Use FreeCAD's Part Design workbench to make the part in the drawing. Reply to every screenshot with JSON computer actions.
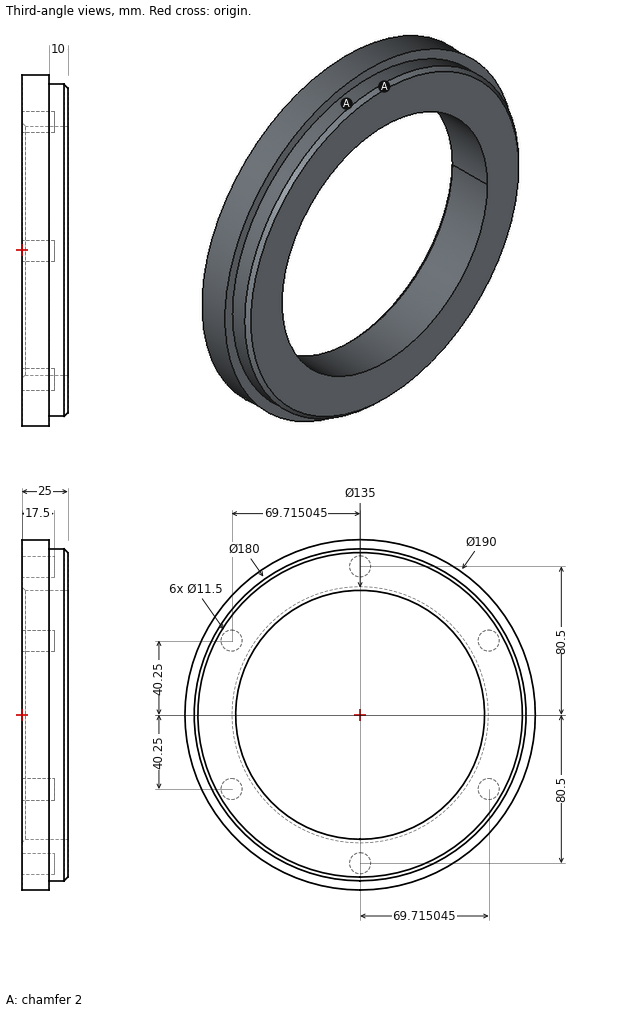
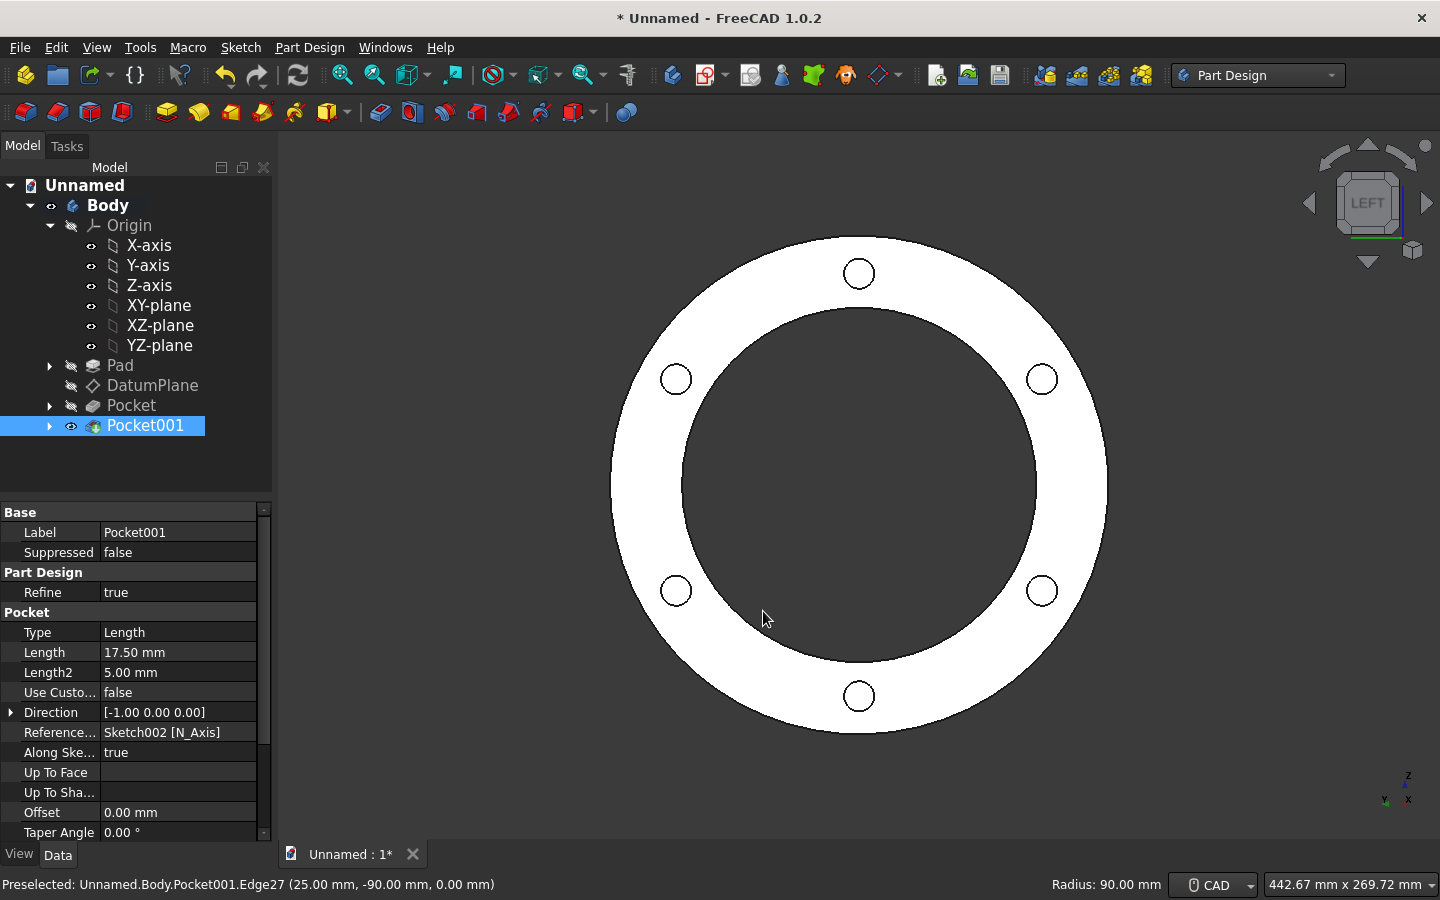
{"action": "left_click", "coordinate": [1036, 484], "text": "ctrl"}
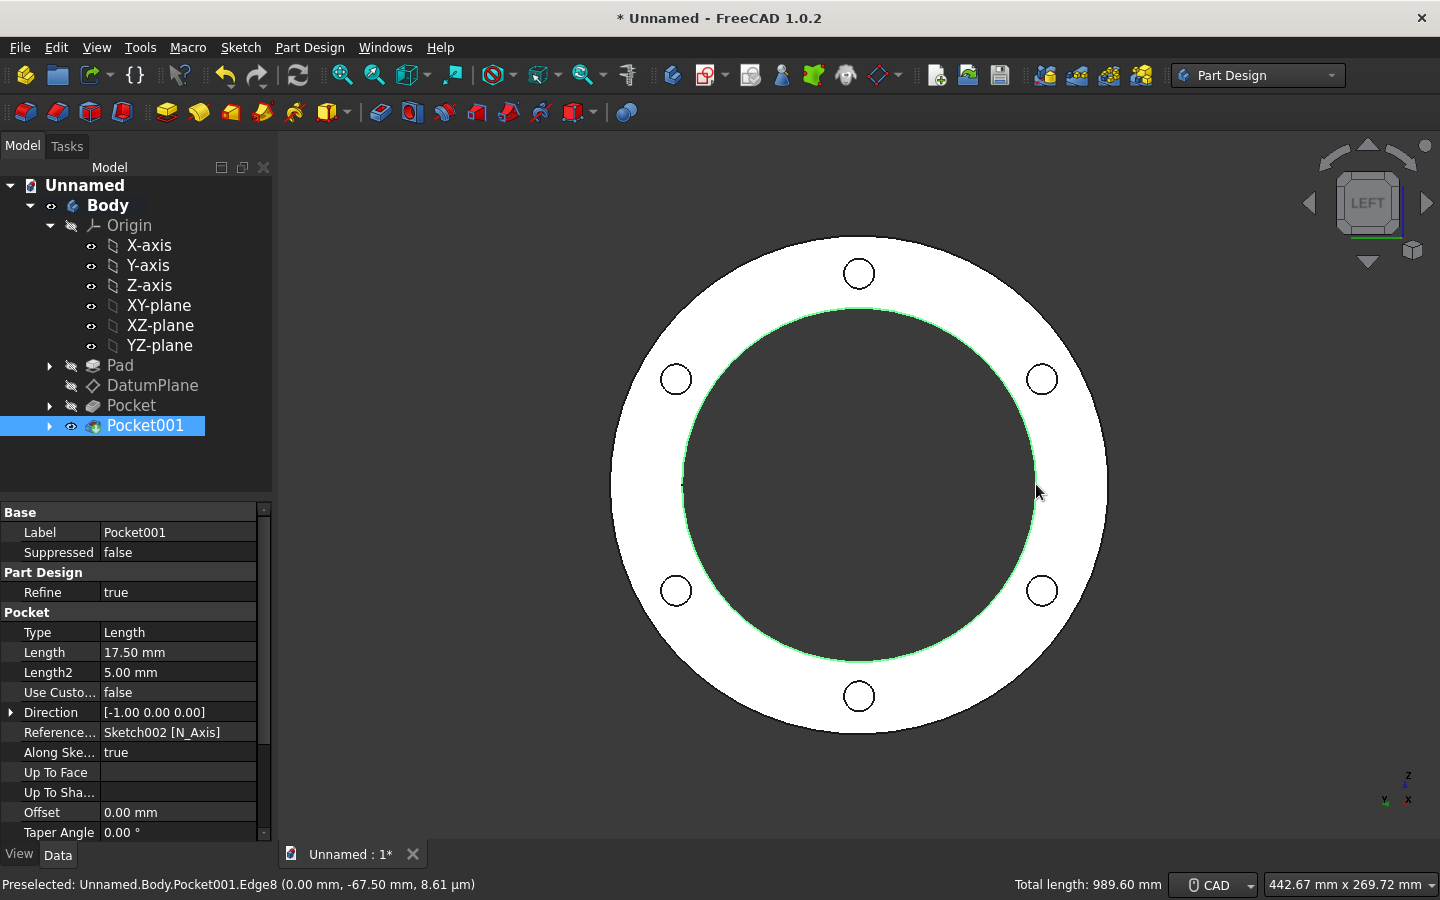
{"action": "left_click", "coordinate": [58, 112]}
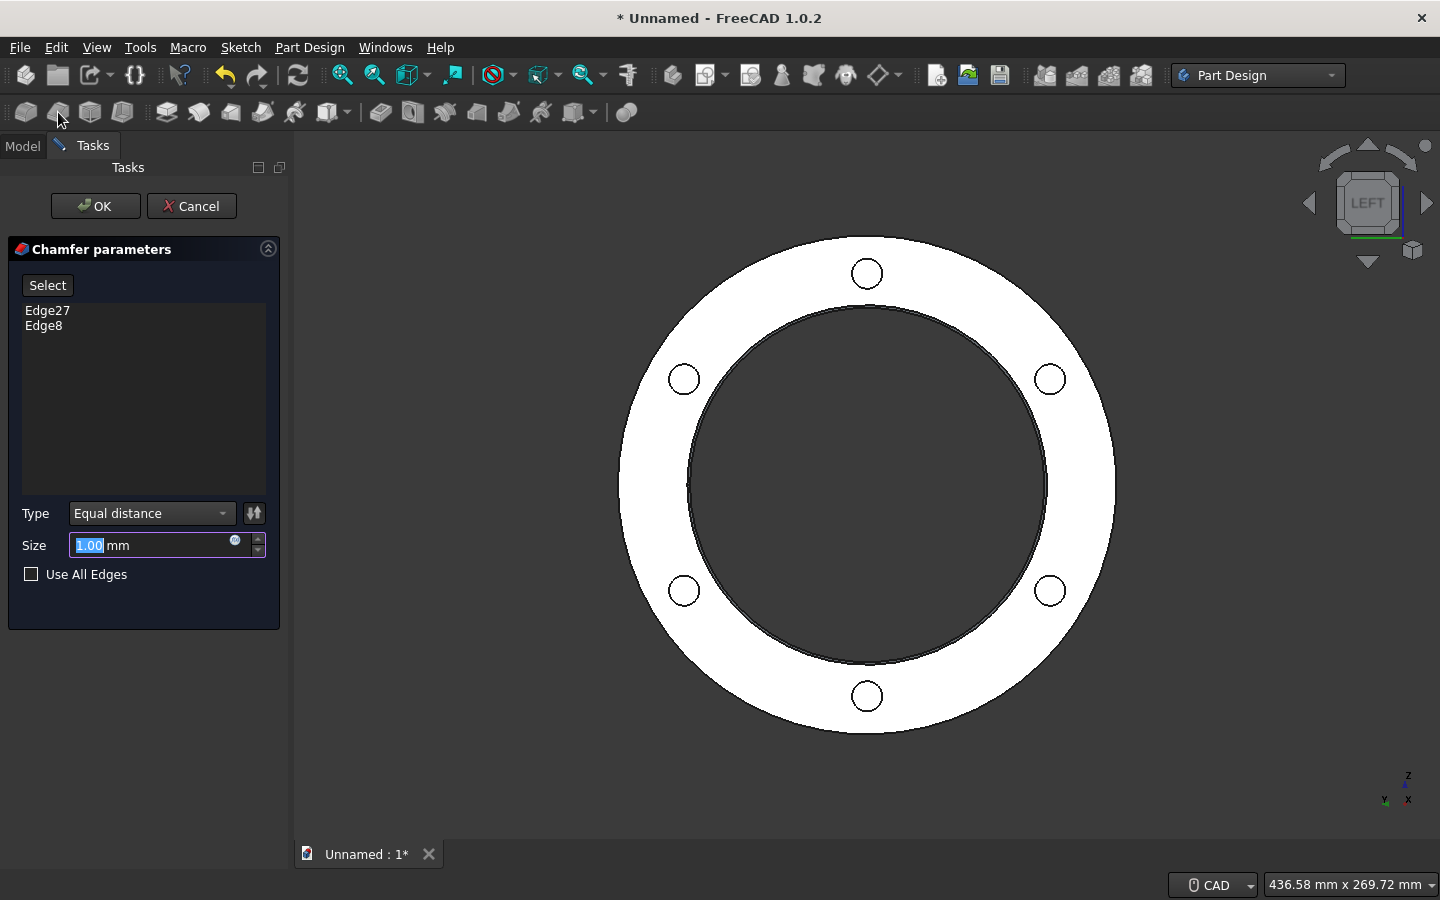
{"action": "type", "text": "2"}
{"action": "key", "text": "Tab"}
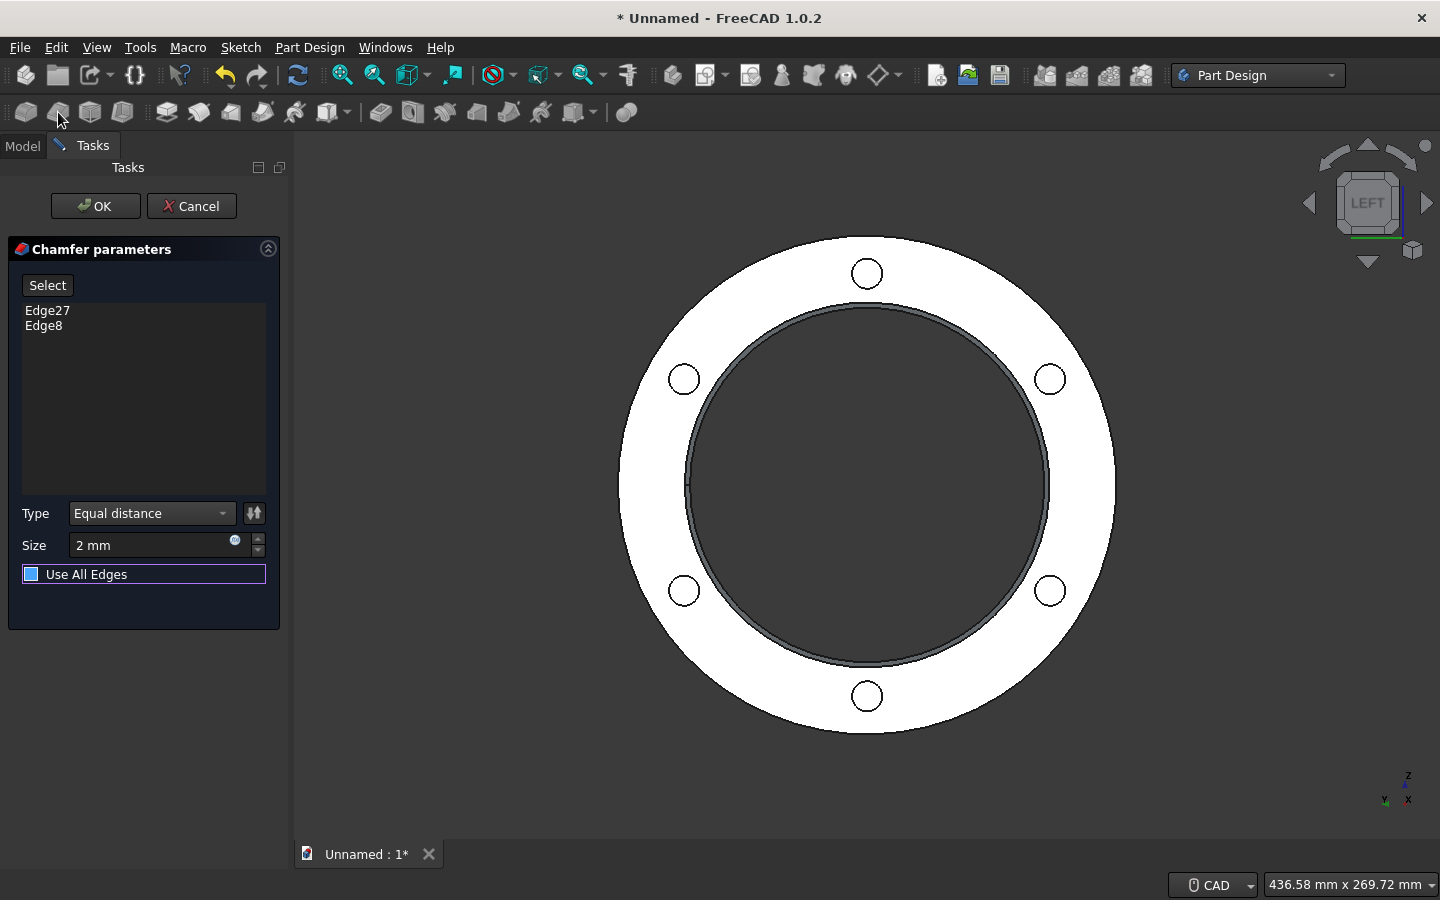
{"action": "left_click", "coordinate": [96, 206]}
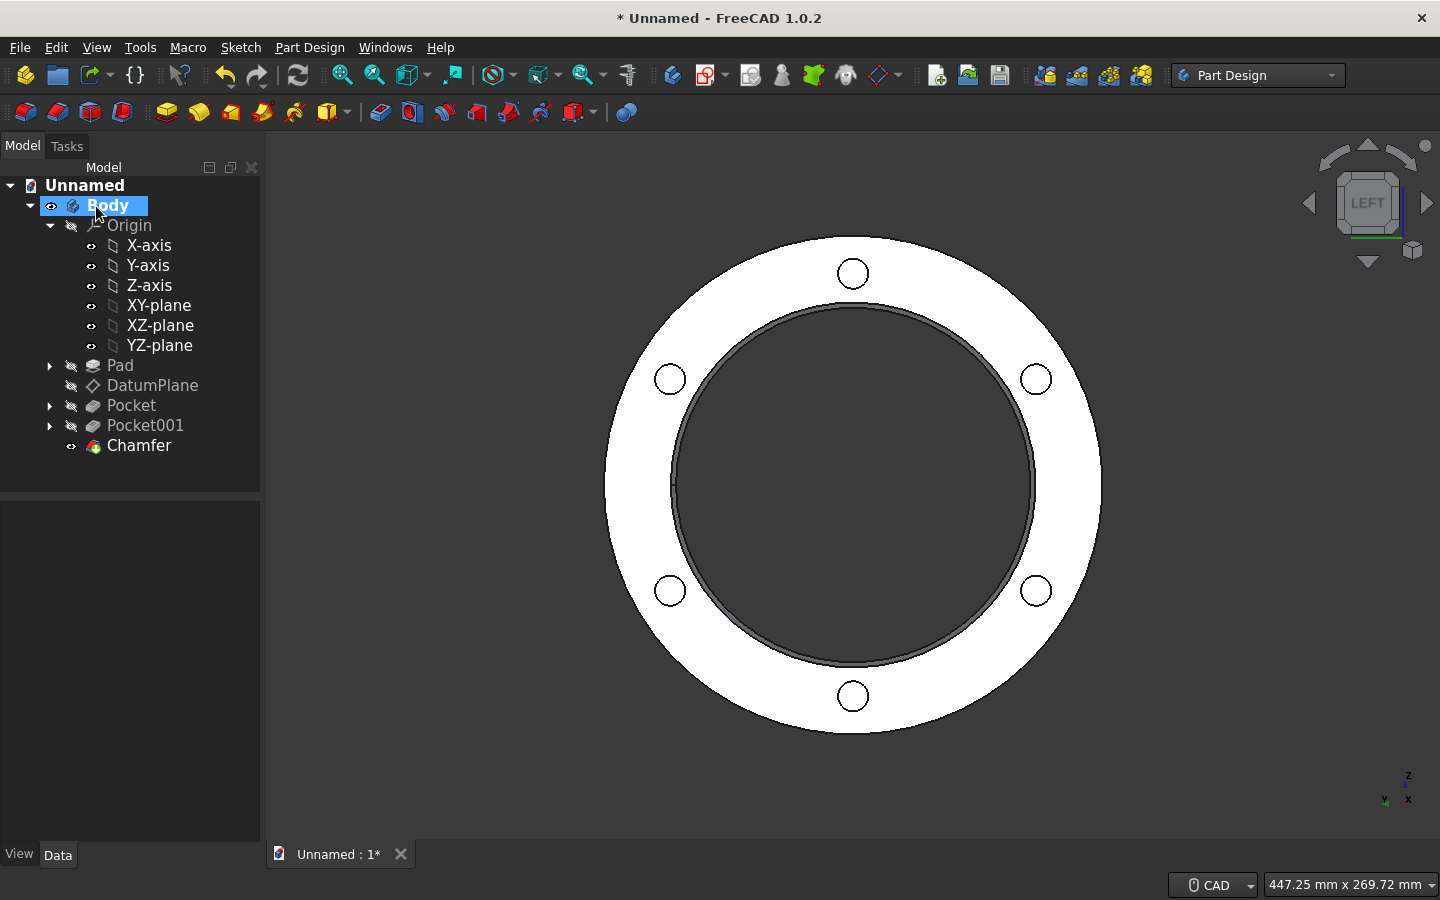
{"action": "key", "text": "0"}